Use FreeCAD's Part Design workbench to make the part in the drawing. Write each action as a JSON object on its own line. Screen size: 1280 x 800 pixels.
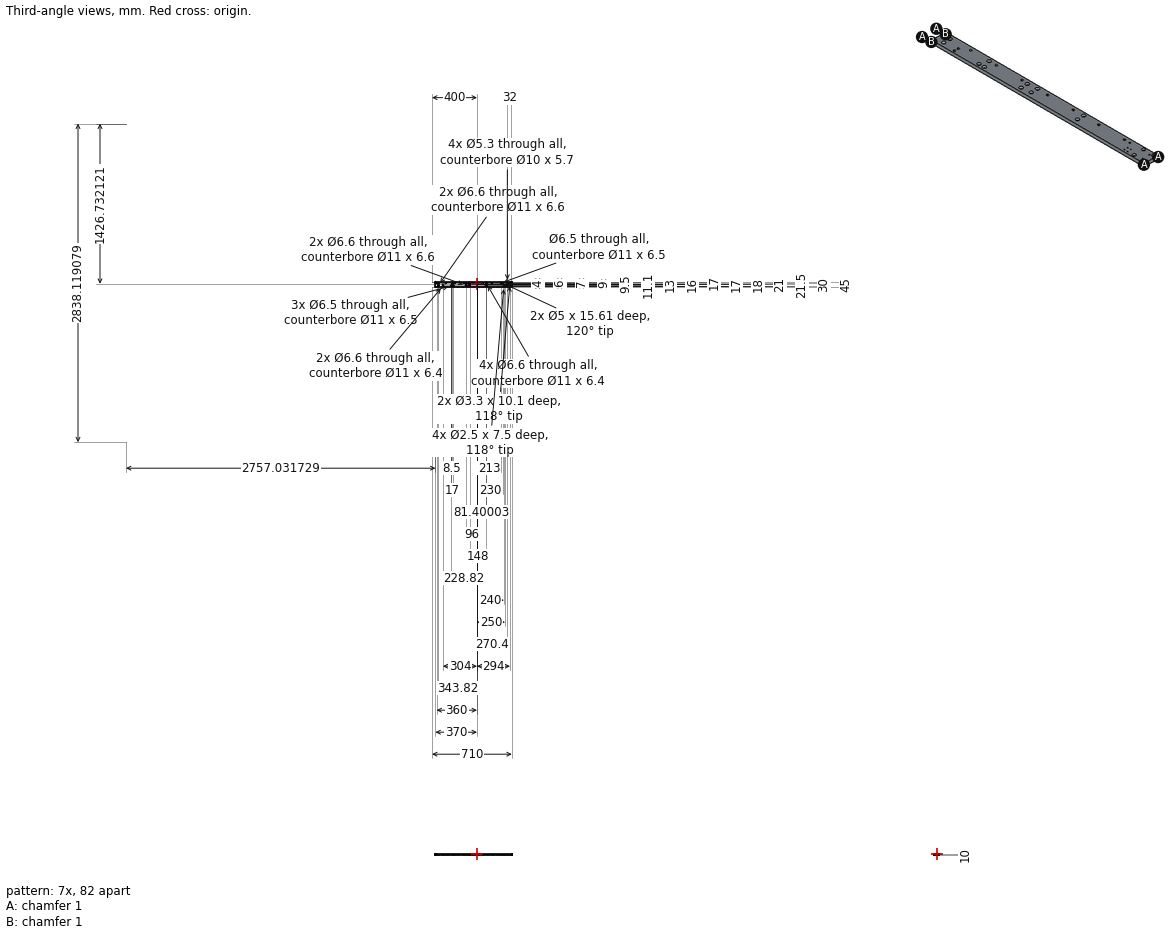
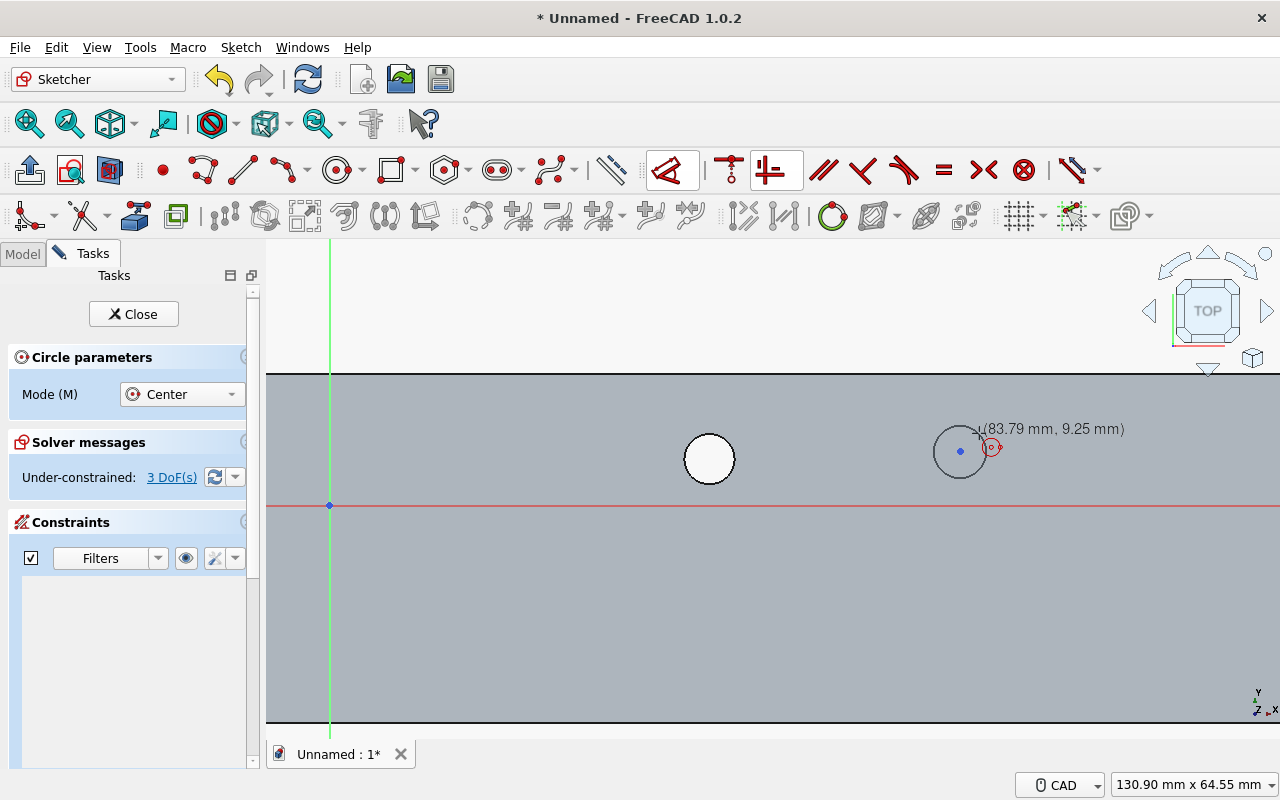
{"action": "left_click", "coordinate": [960, 606]}
{"action": "left_click", "coordinate": [979, 588]}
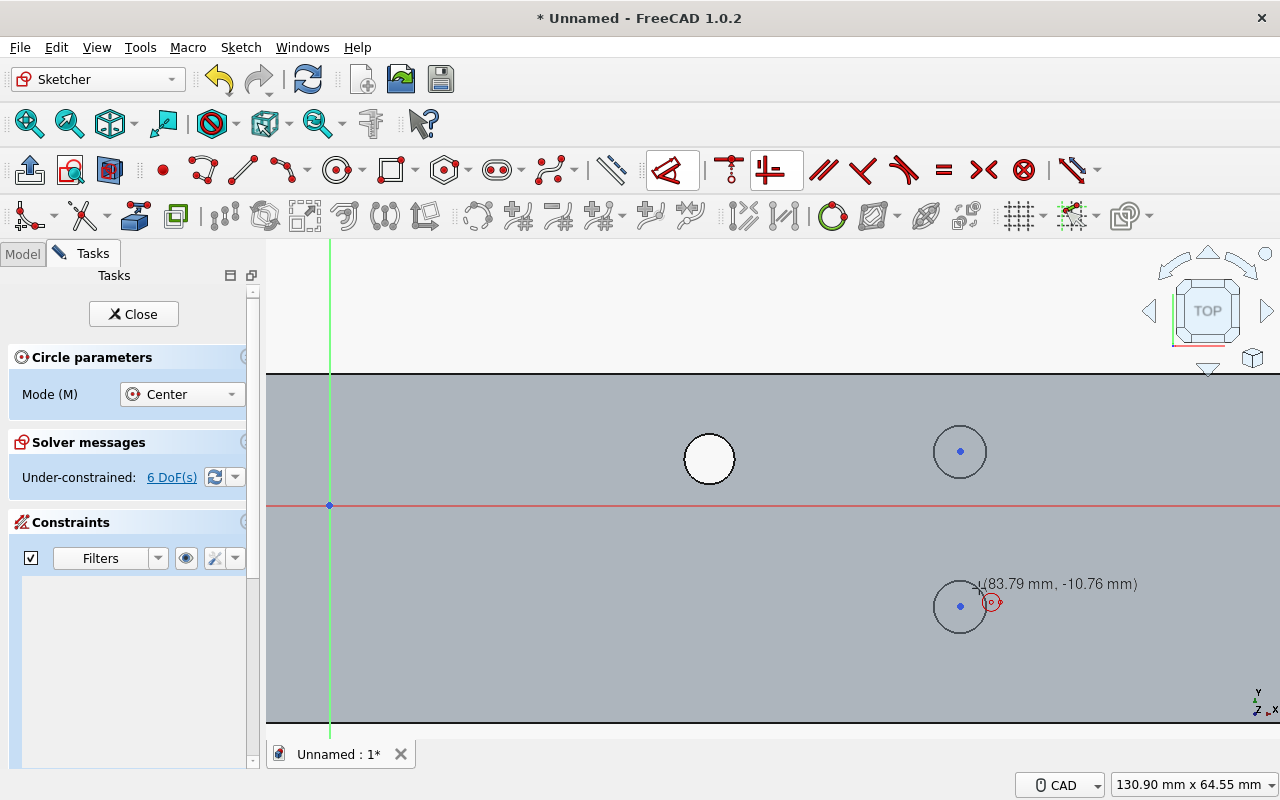
{"action": "scroll", "coordinate": [963, 456], "scroll_direction": "down", "scroll_amount": 4}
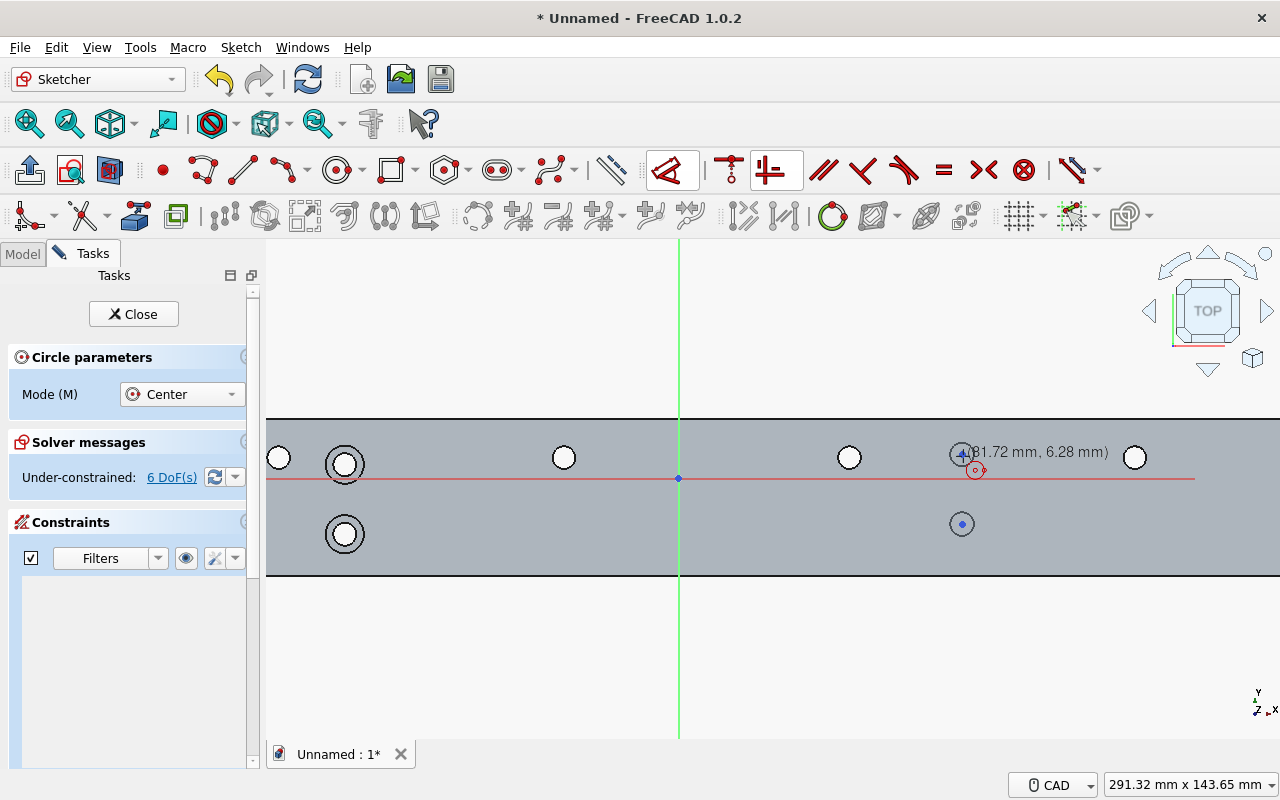
{"action": "scroll", "coordinate": [447, 454], "scroll_direction": "up", "scroll_amount": 4}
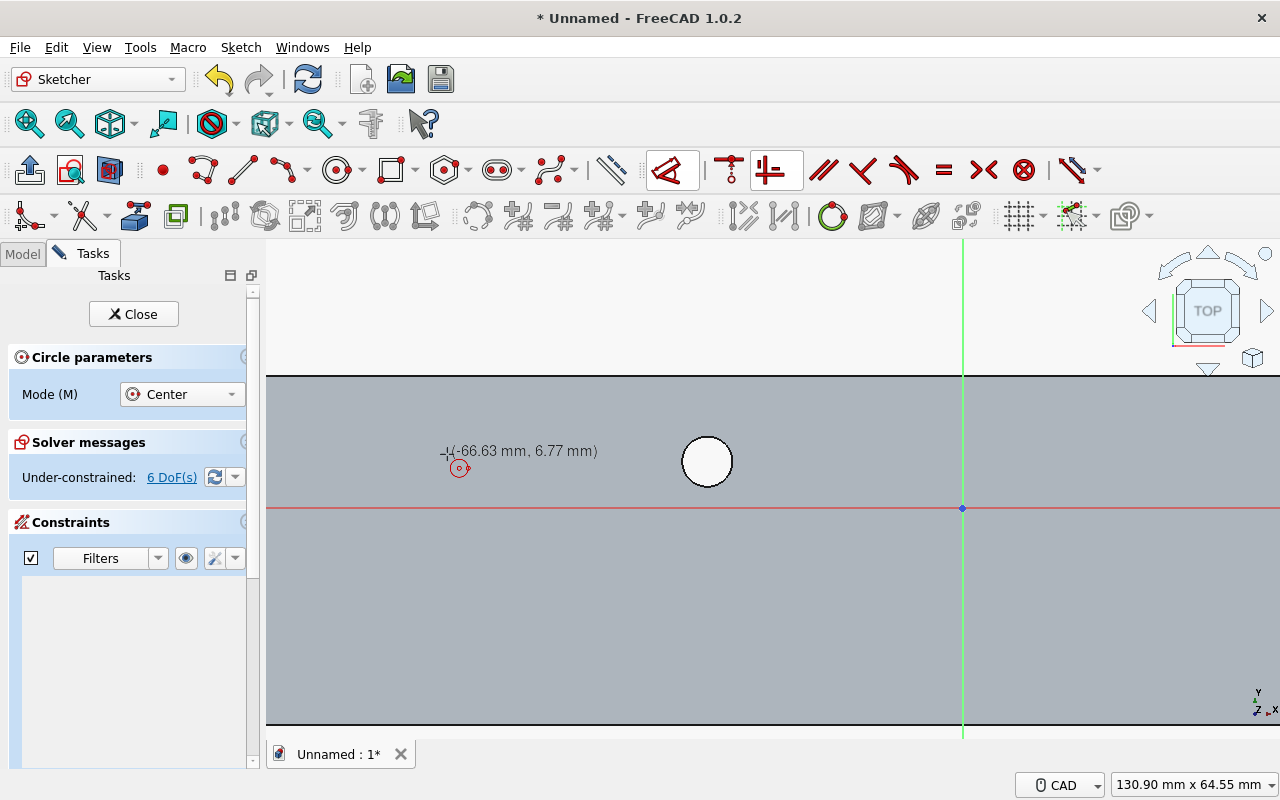
{"action": "left_click", "coordinate": [447, 454]}
{"action": "left_click", "coordinate": [465, 436]}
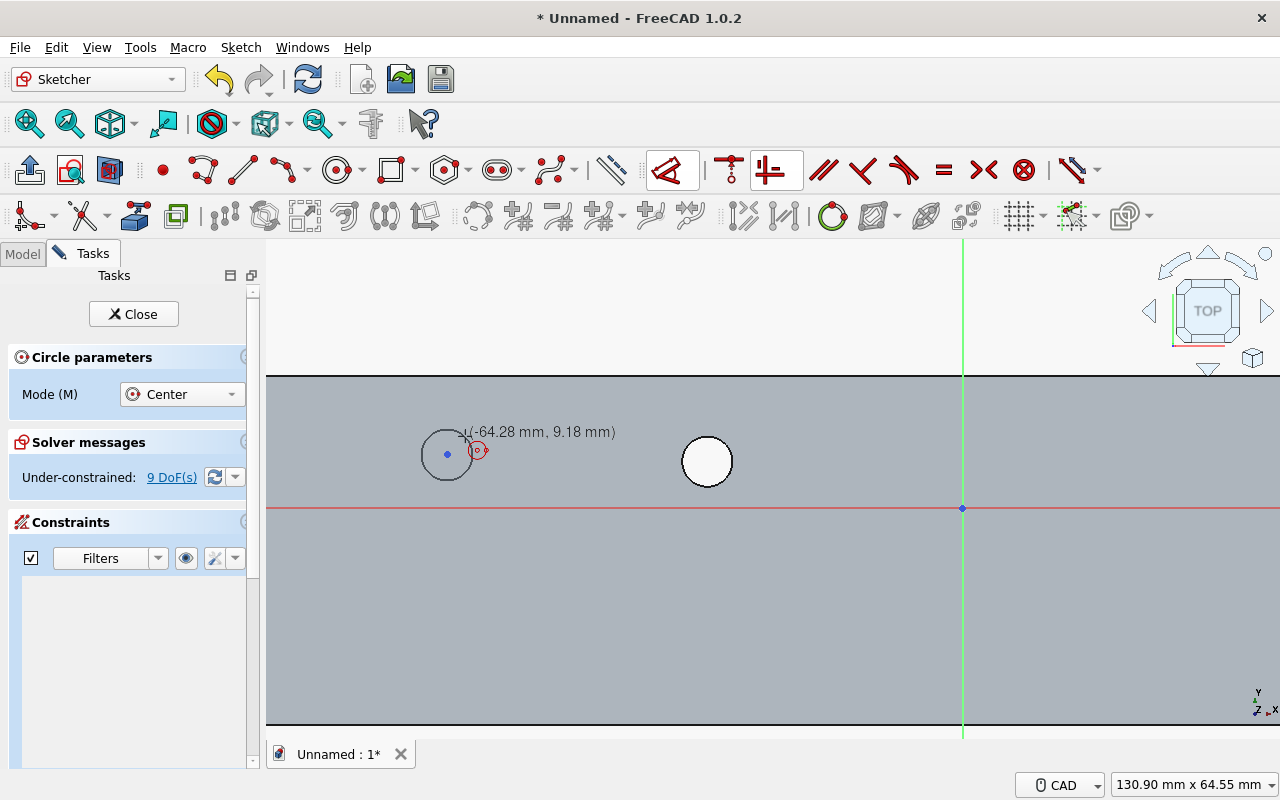
{"action": "left_click", "coordinate": [447, 609]}
{"action": "left_click", "coordinate": [465, 591]}
{"action": "key", "text": "Escape"}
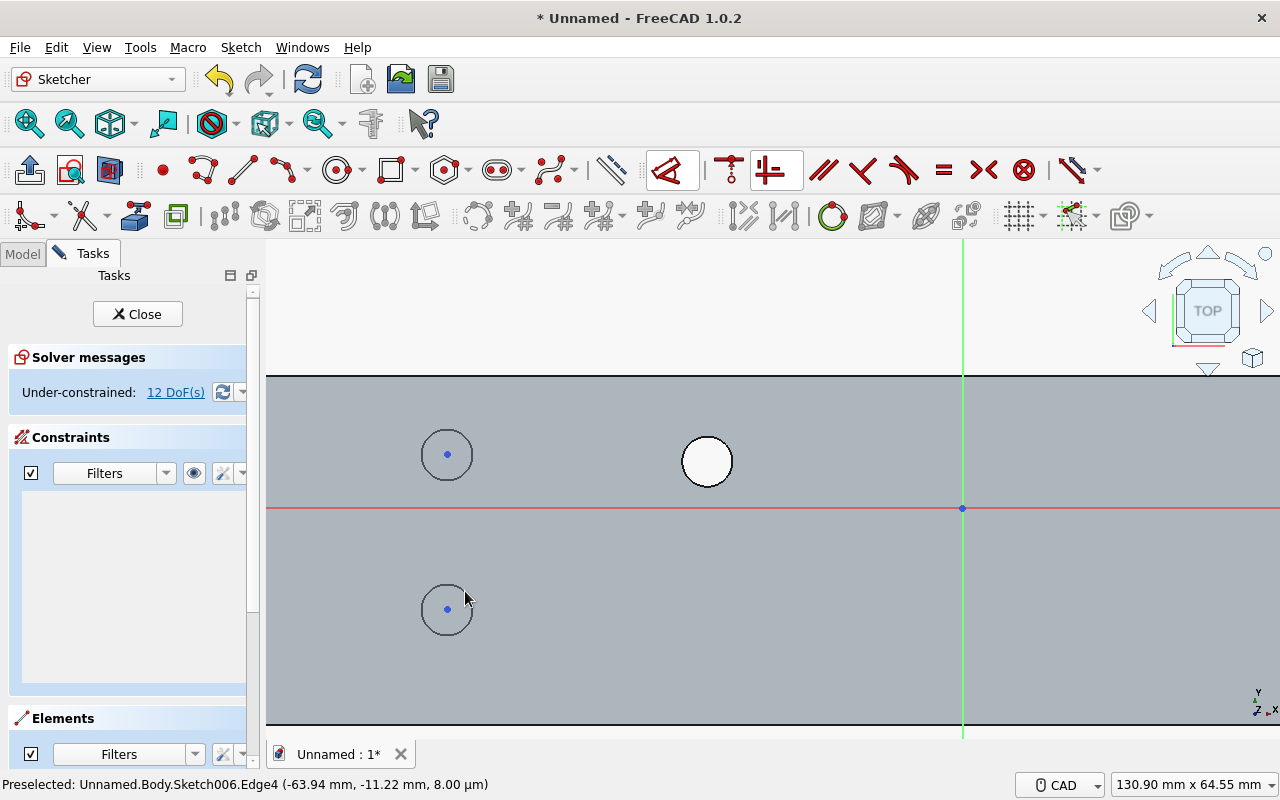
{"action": "scroll", "coordinate": [447, 454], "scroll_direction": "down", "scroll_amount": 4}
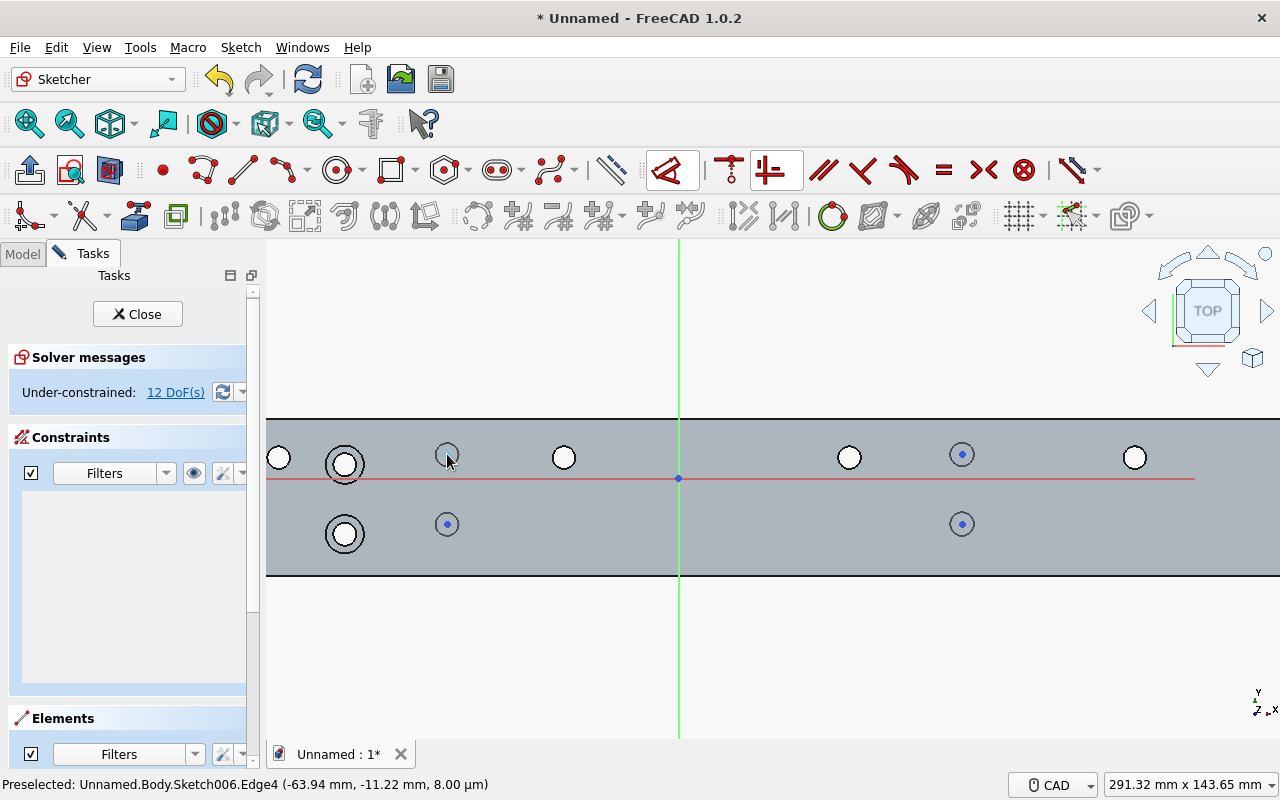
{"action": "left_click", "coordinate": [970, 446]}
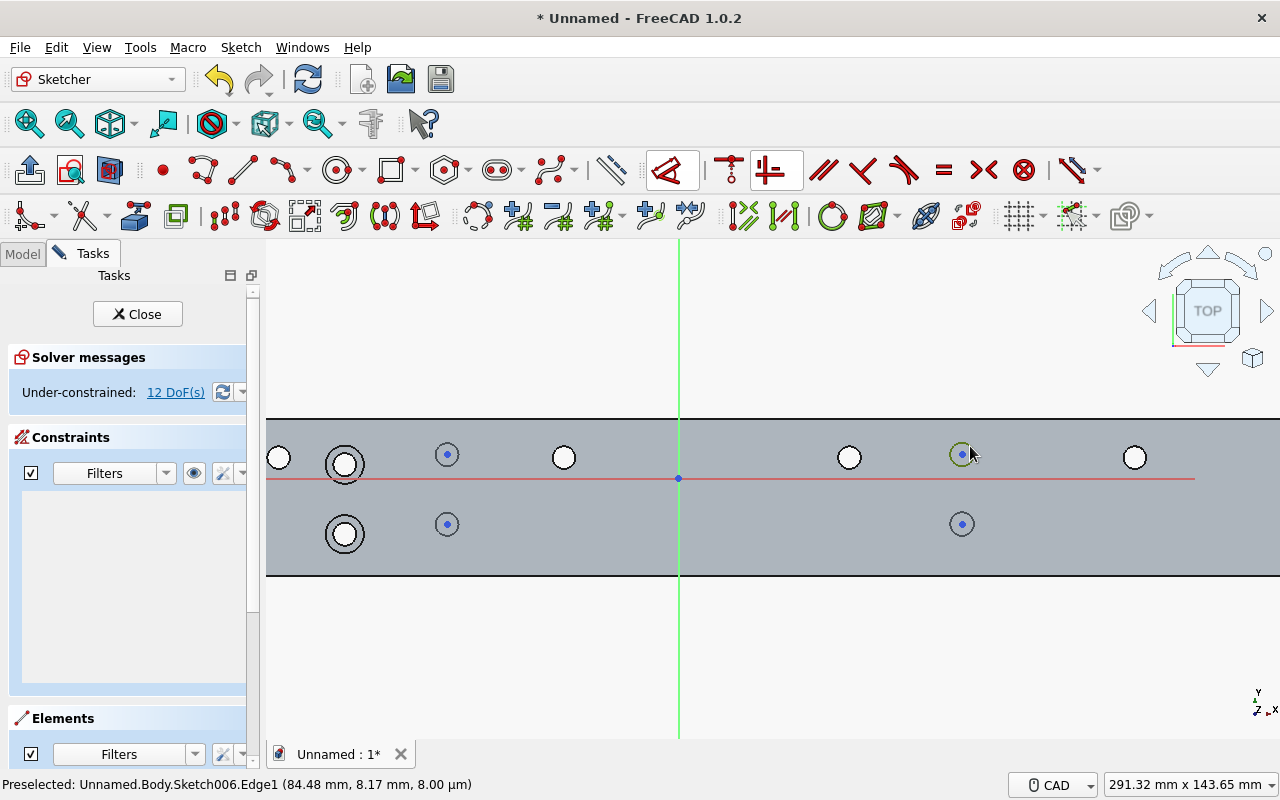
{"action": "left_click", "coordinate": [970, 516]}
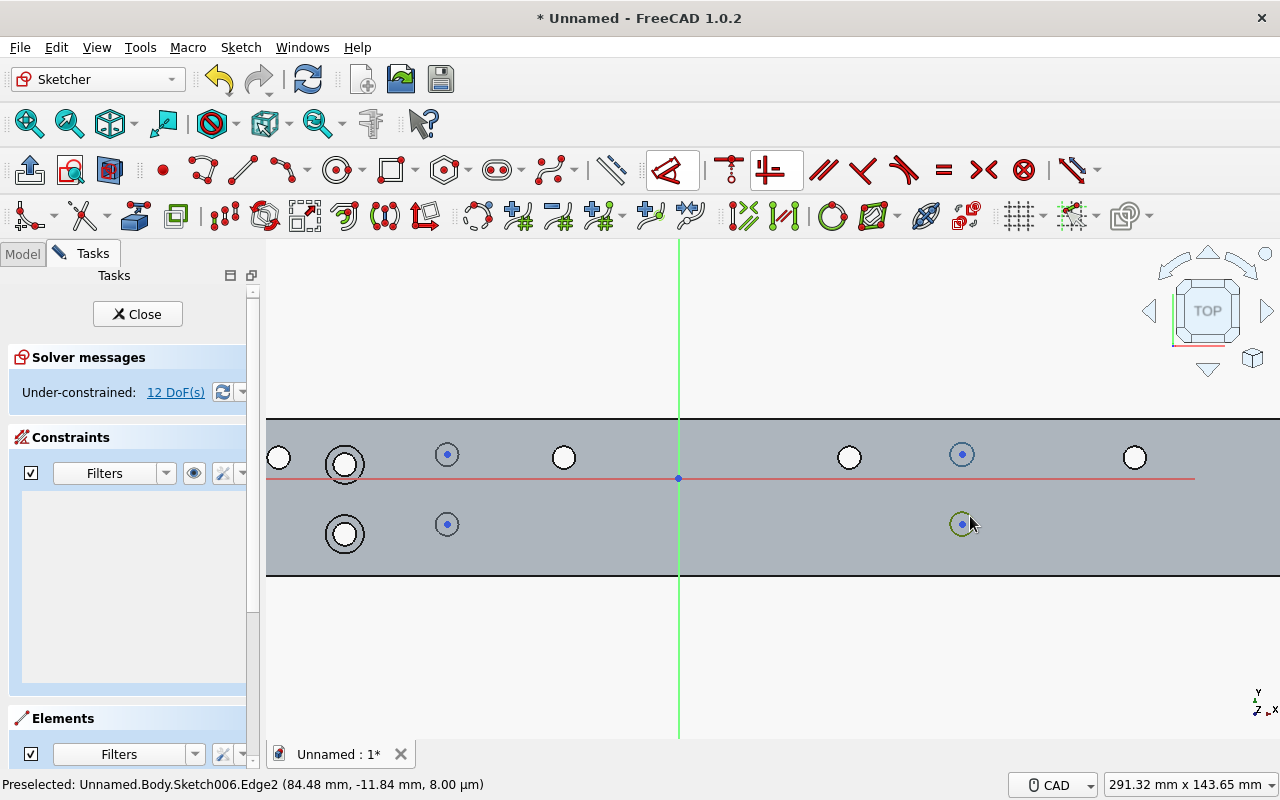
{"action": "left_click", "coordinate": [455, 447]}